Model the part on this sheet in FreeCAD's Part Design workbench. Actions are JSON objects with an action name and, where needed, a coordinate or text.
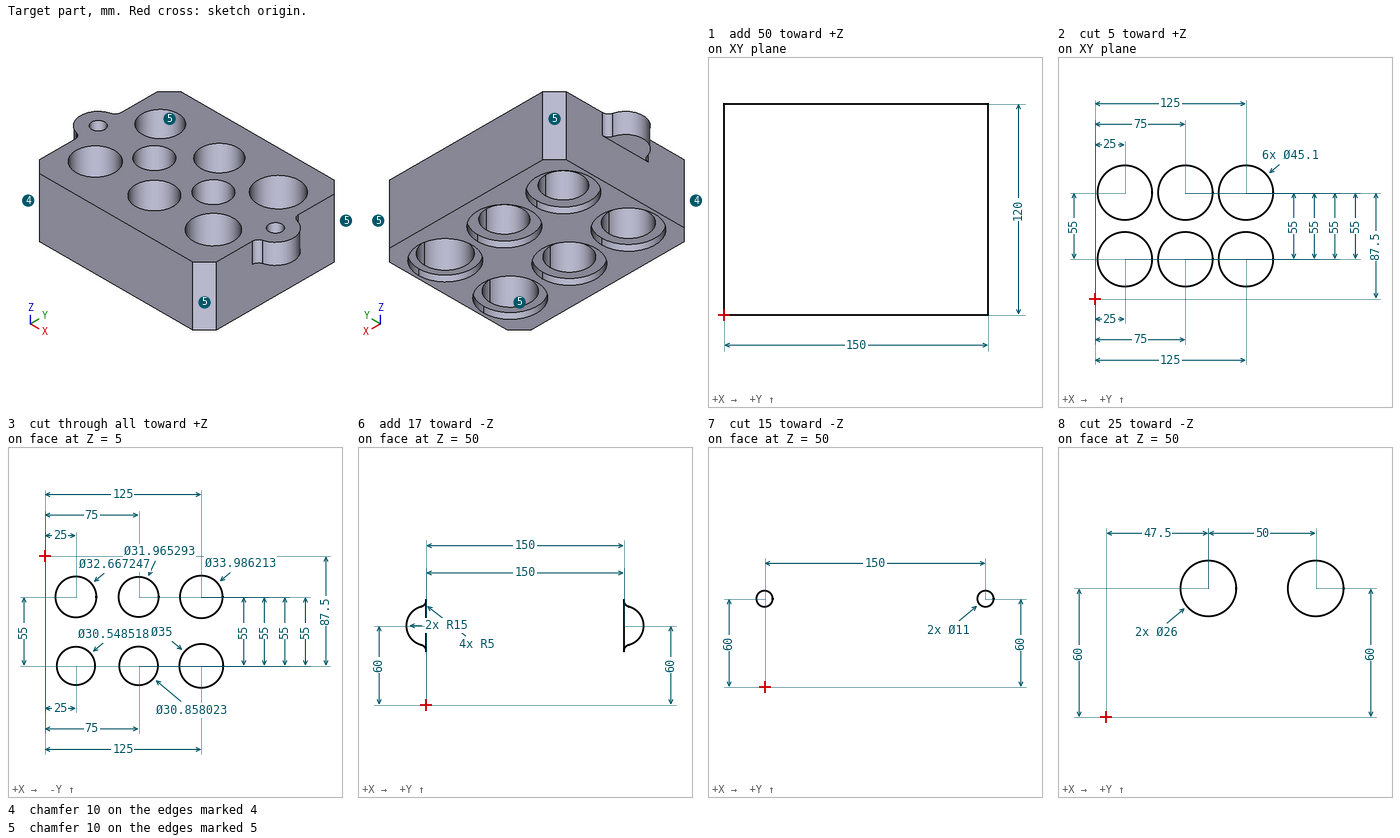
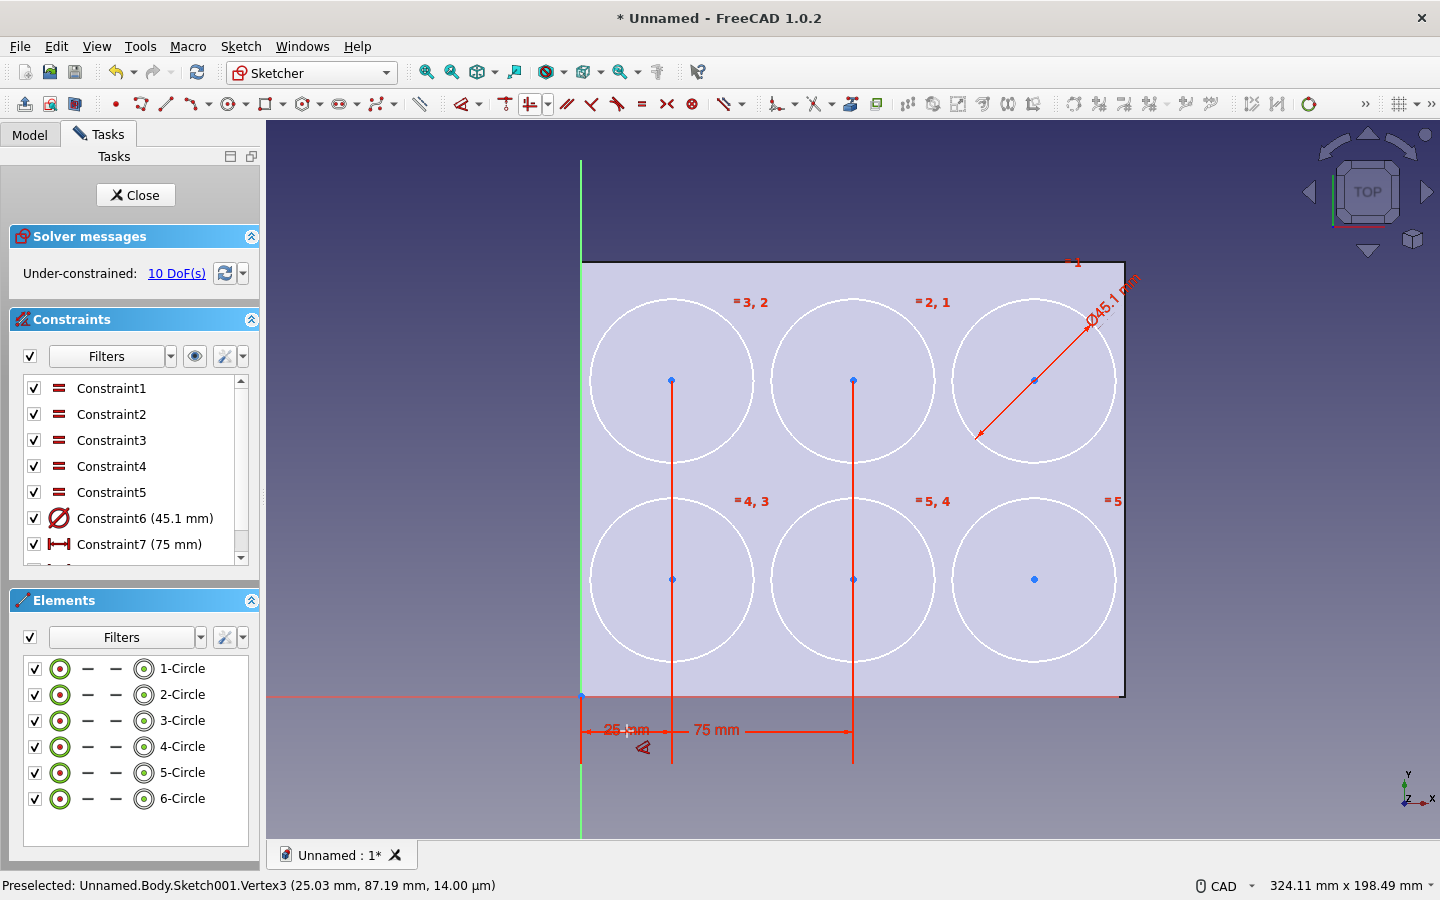
{"action": "left_click", "coordinate": [672, 580]}
{"action": "left_click", "coordinate": [627, 546]}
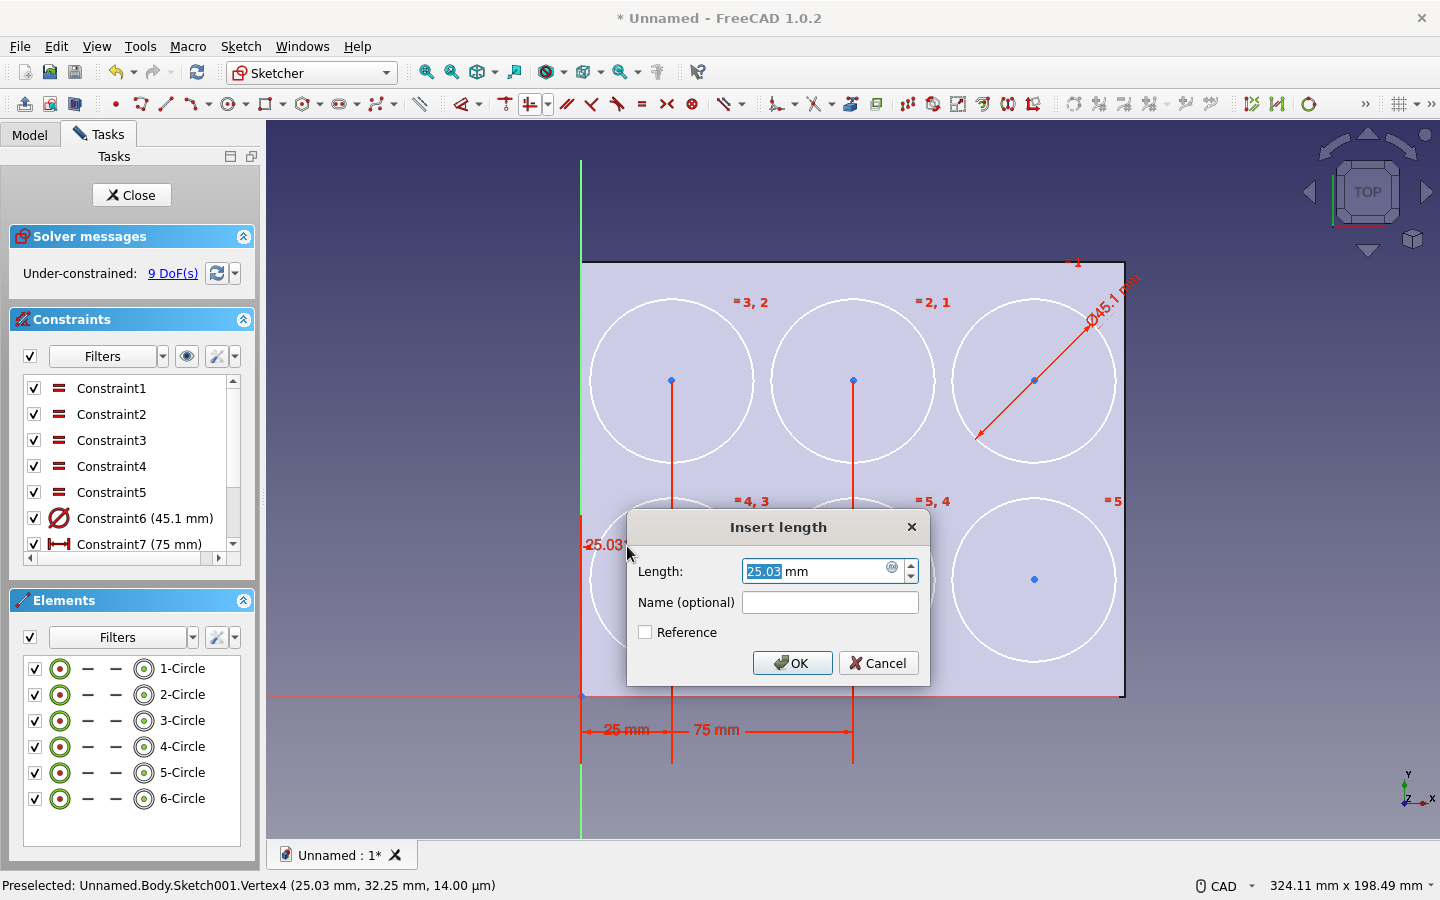
{"action": "type", "text": "25"}
{"action": "key", "text": "Return"}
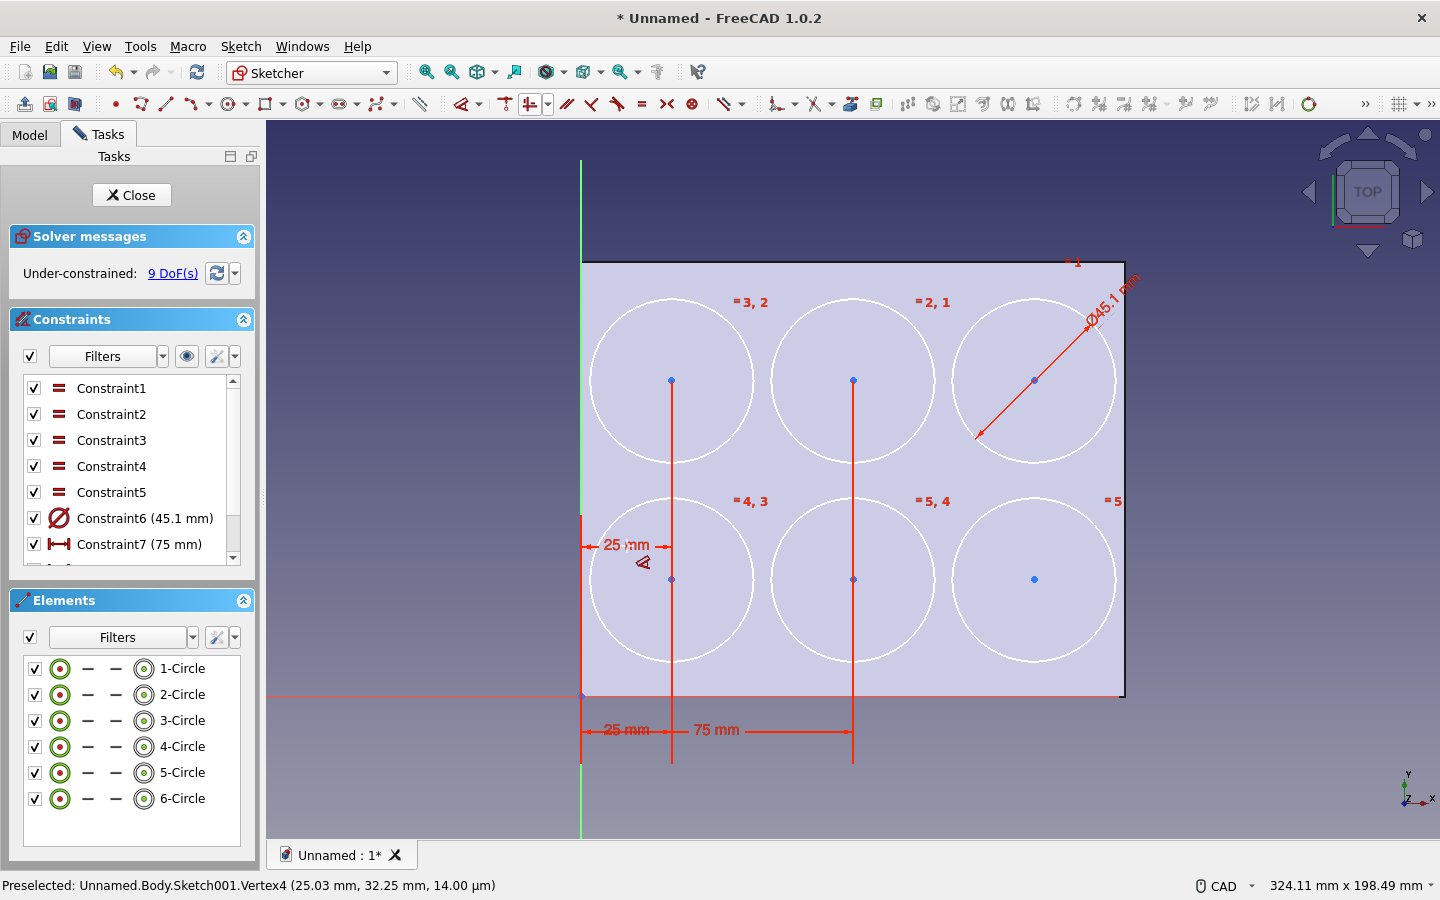
{"action": "left_click", "coordinate": [853, 580]}
{"action": "left_click", "coordinate": [812, 731]}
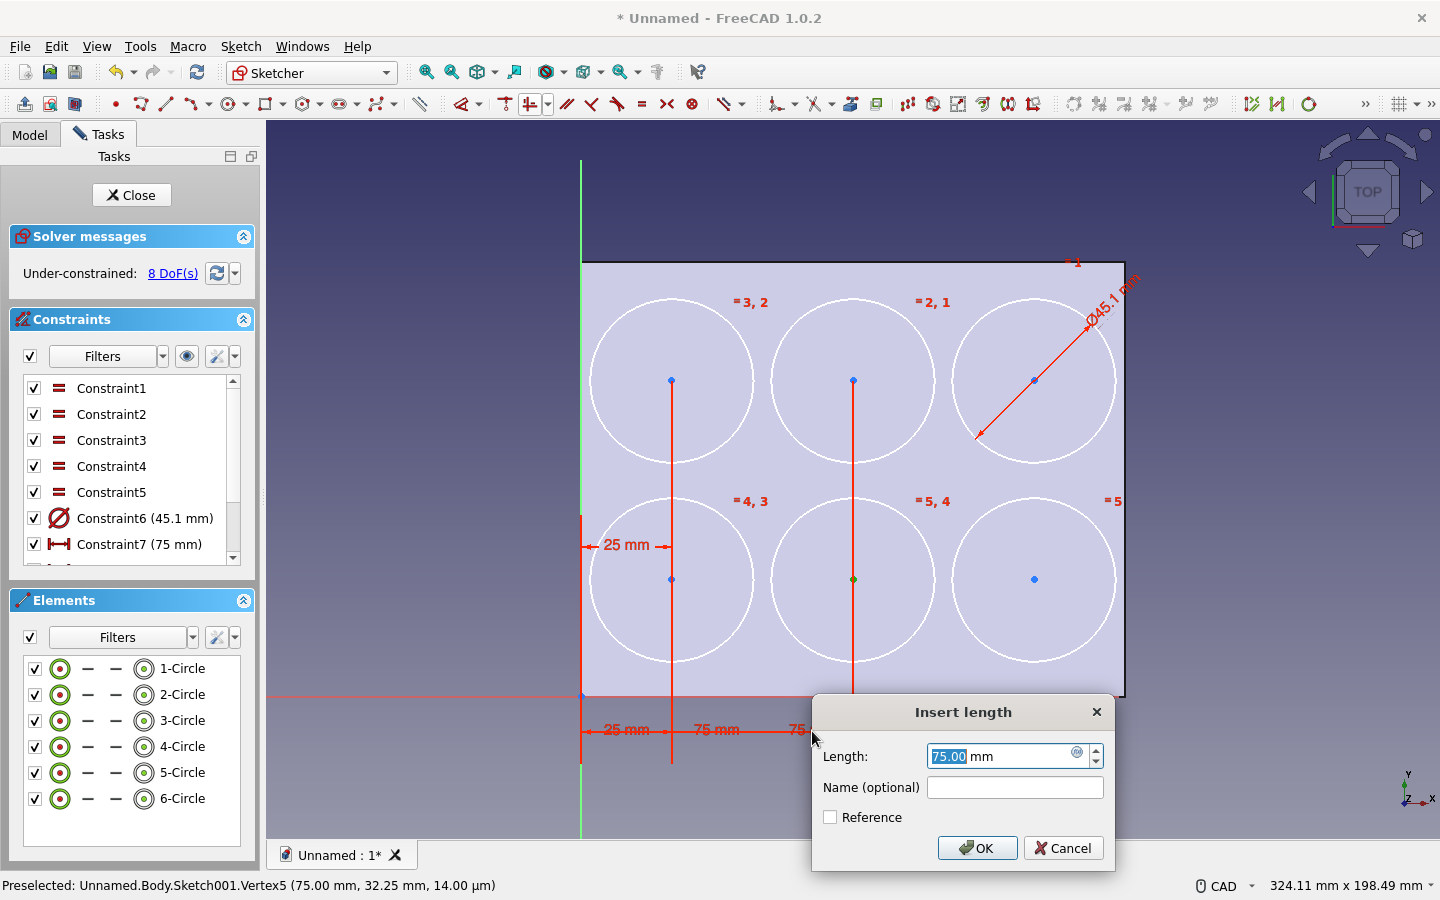
{"action": "type", "text": "75"}
{"action": "key", "text": "Return"}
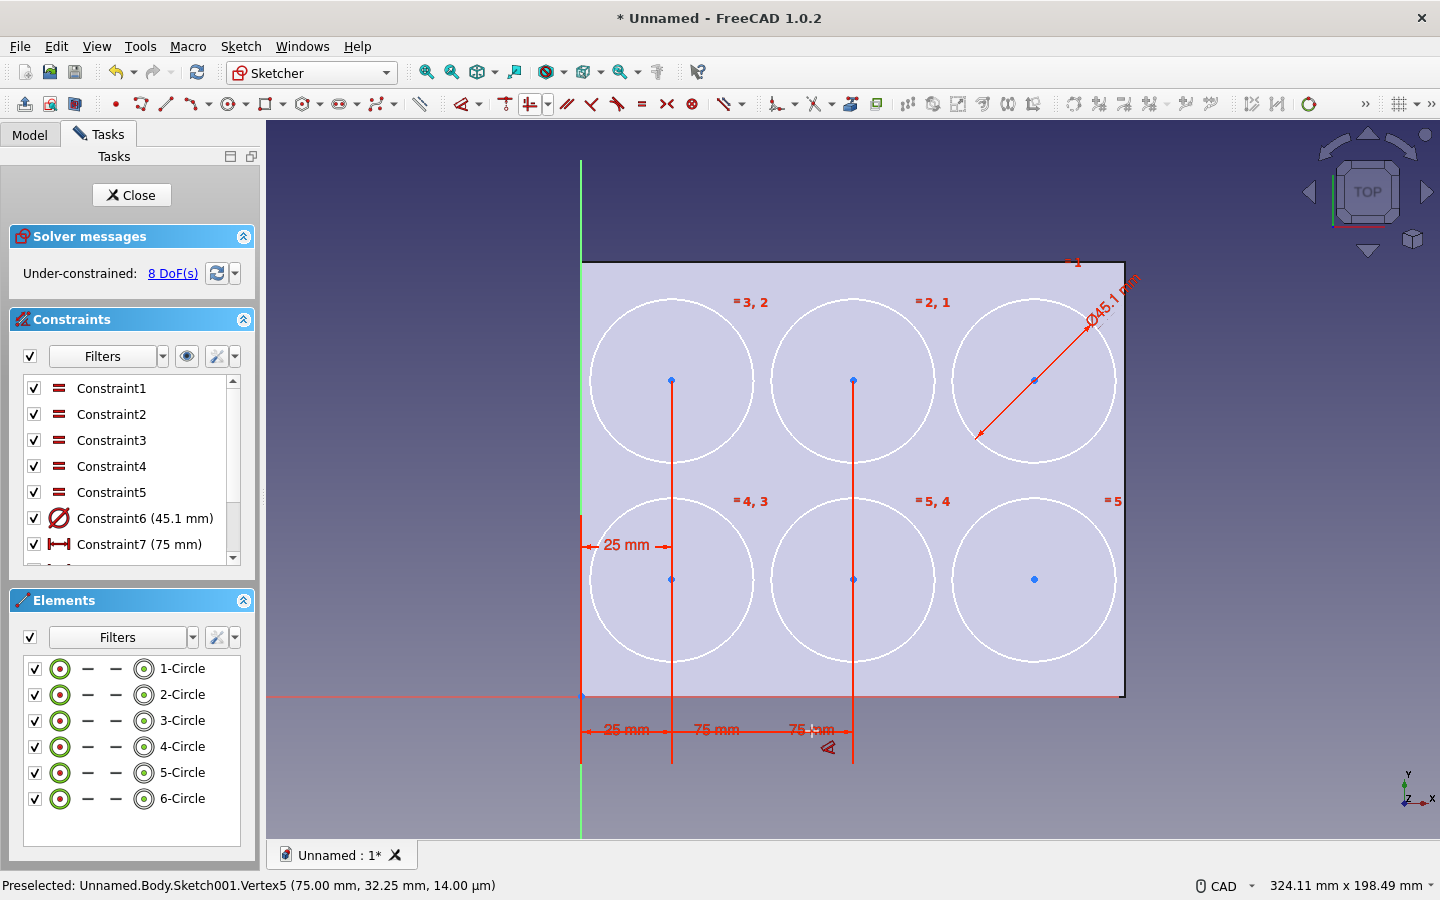
{"action": "left_click", "coordinate": [1034, 381]}
{"action": "left_click", "coordinate": [912, 731]}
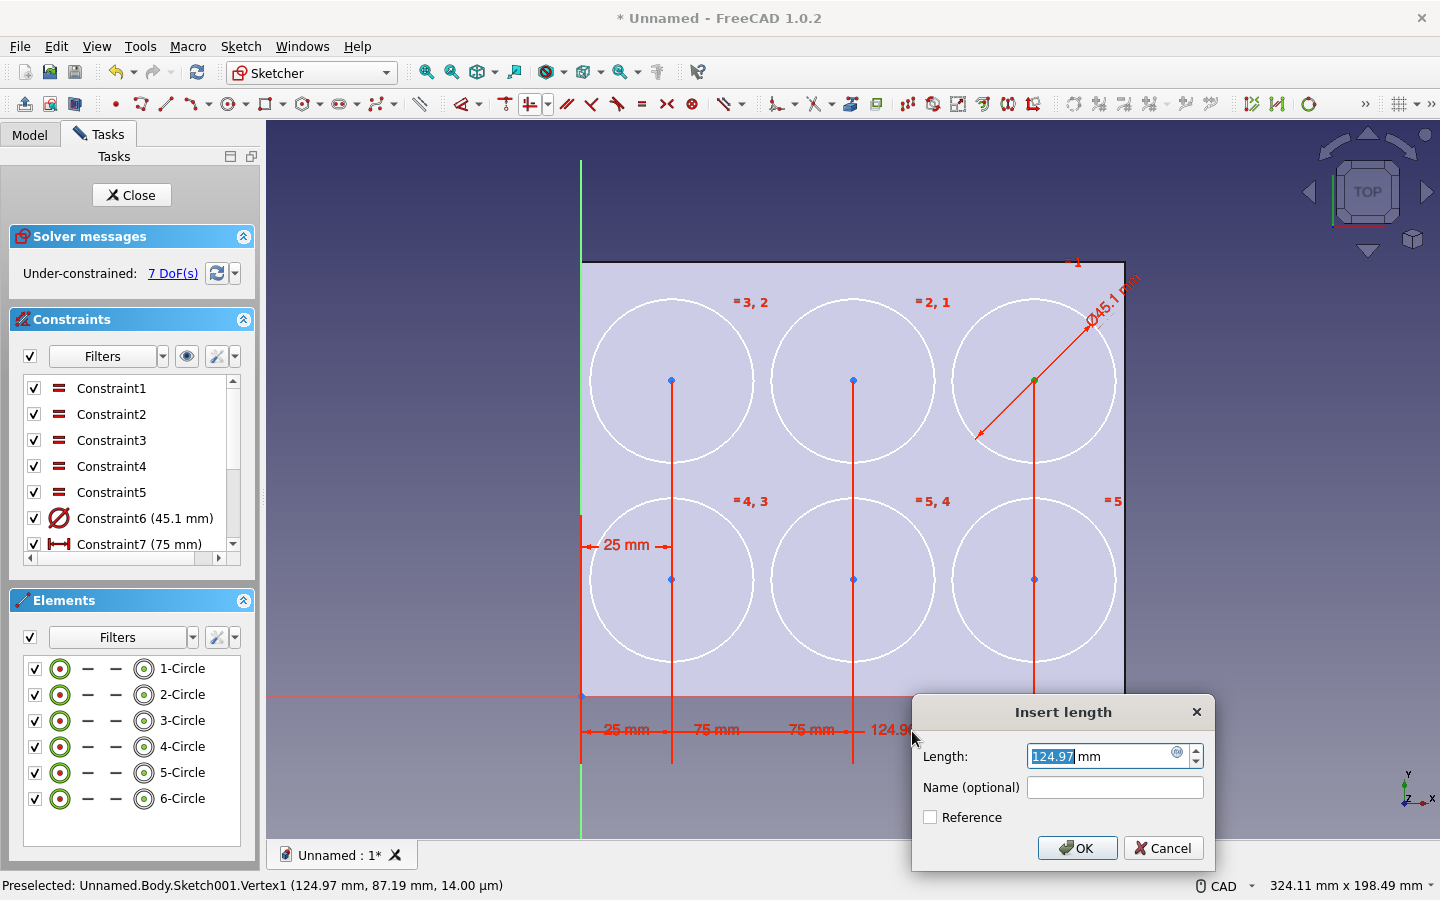
{"action": "type", "text": "125"}
{"action": "key", "text": "Return"}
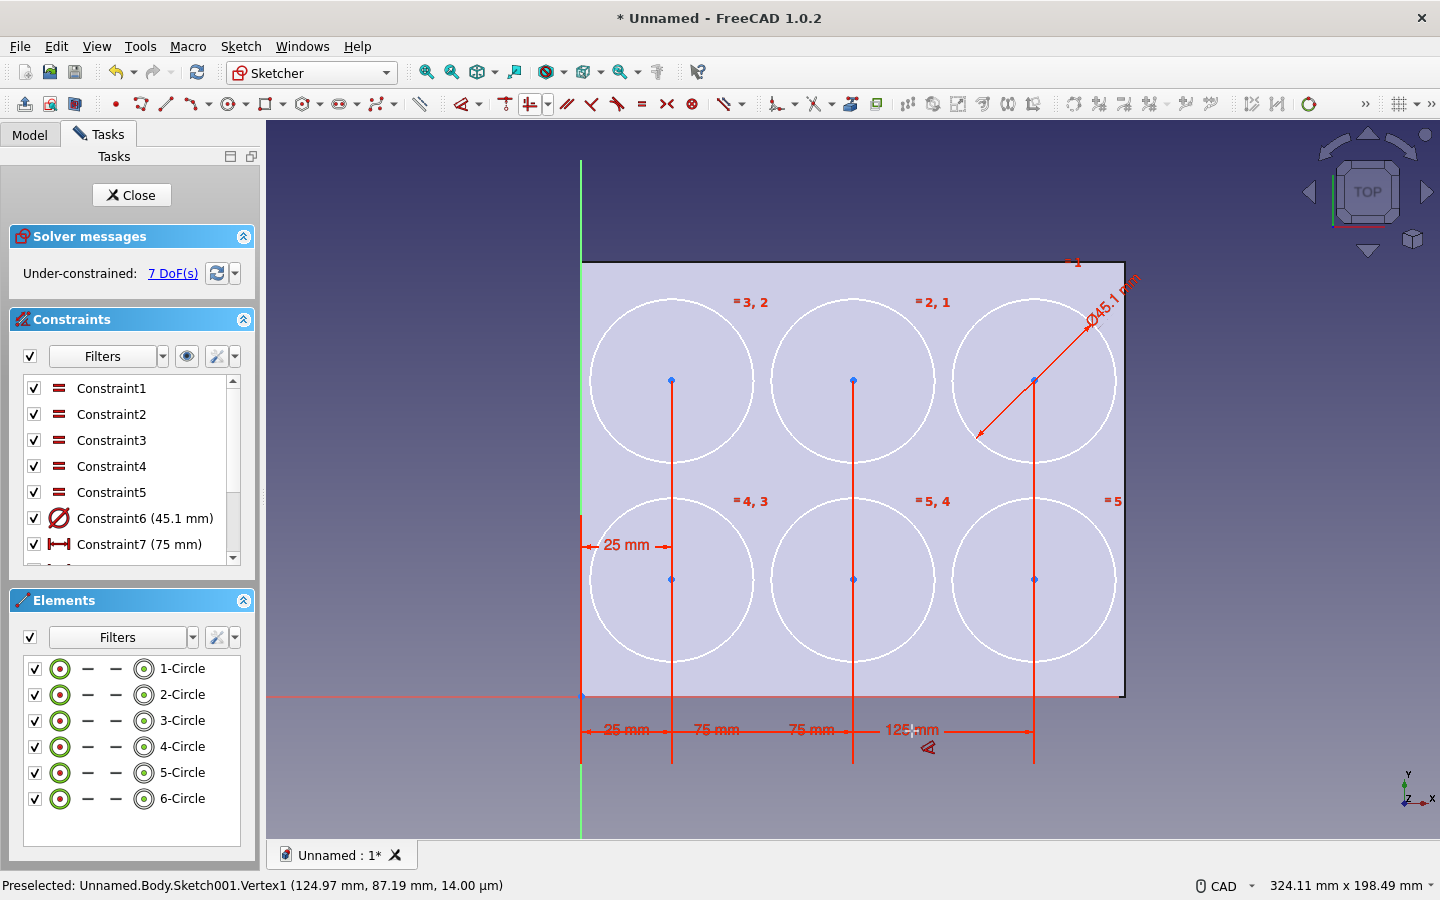
{"action": "left_click", "coordinate": [1034, 580]}
{"action": "left_click", "coordinate": [808, 546]}